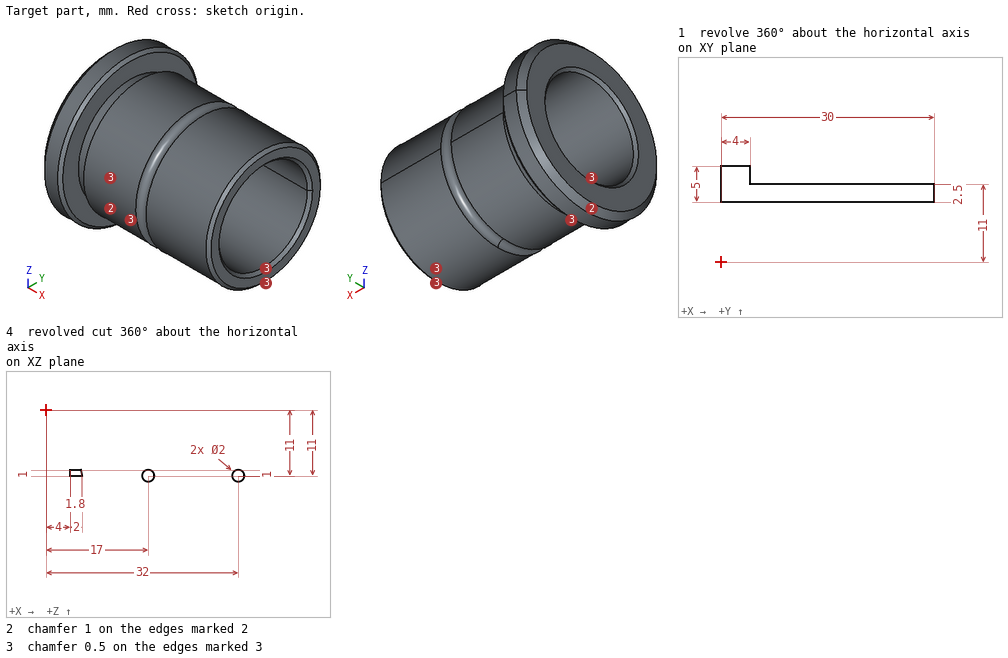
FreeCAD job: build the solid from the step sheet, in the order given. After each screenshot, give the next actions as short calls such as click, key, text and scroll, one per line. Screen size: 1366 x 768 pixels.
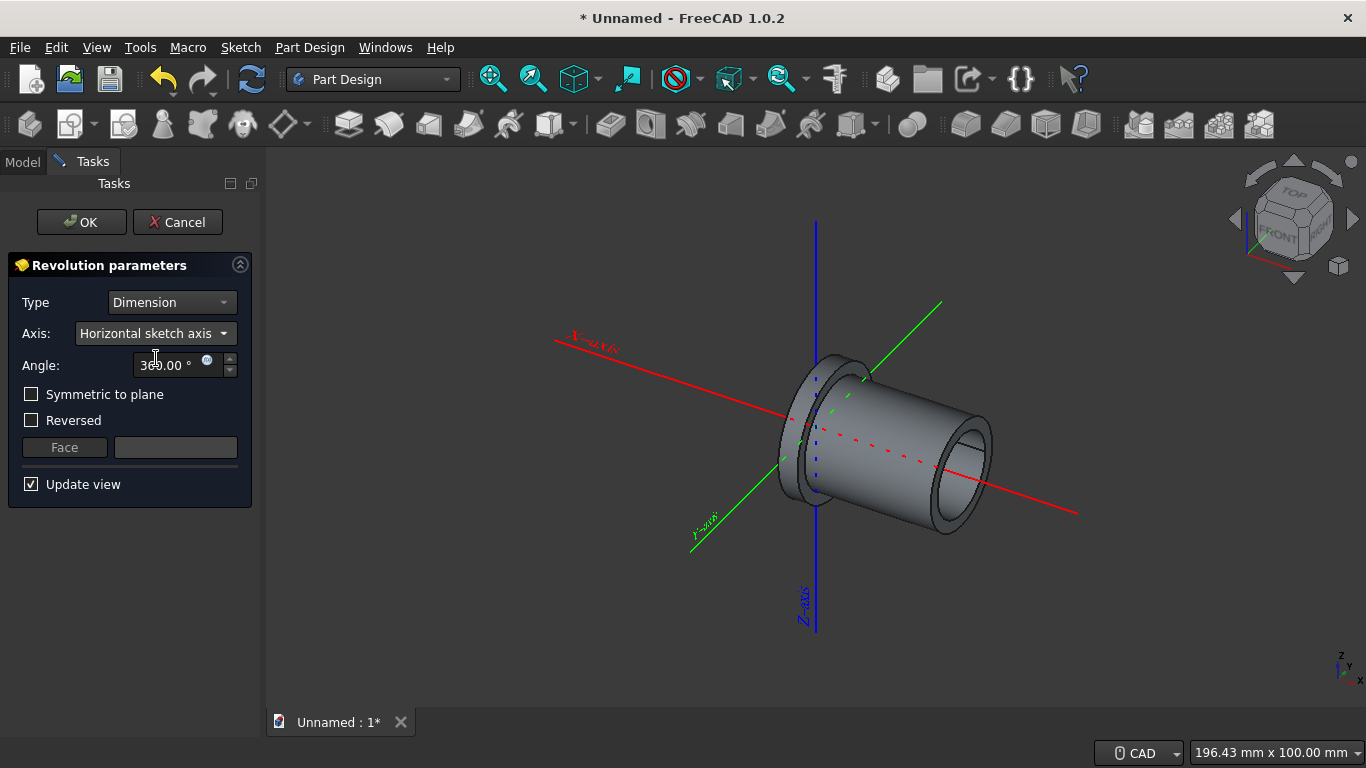
click(82, 222)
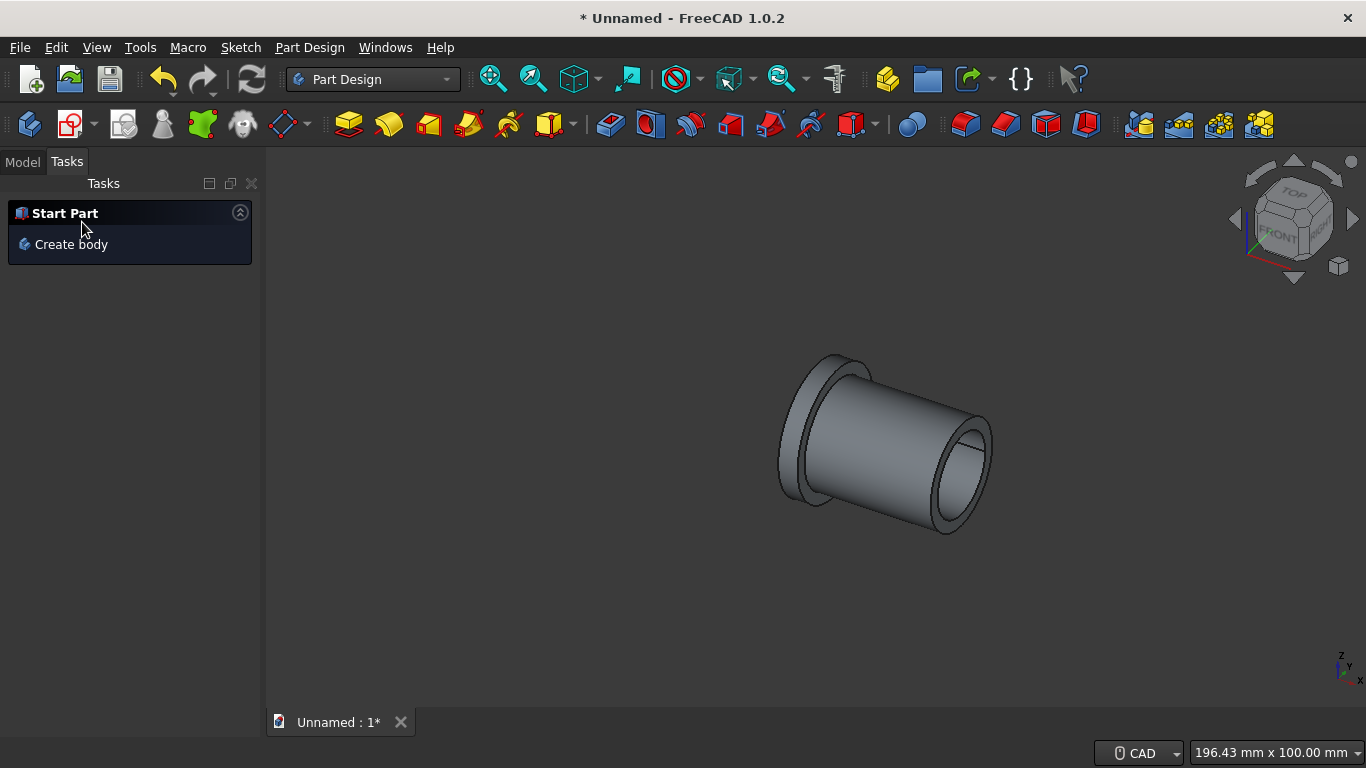
click(494, 80)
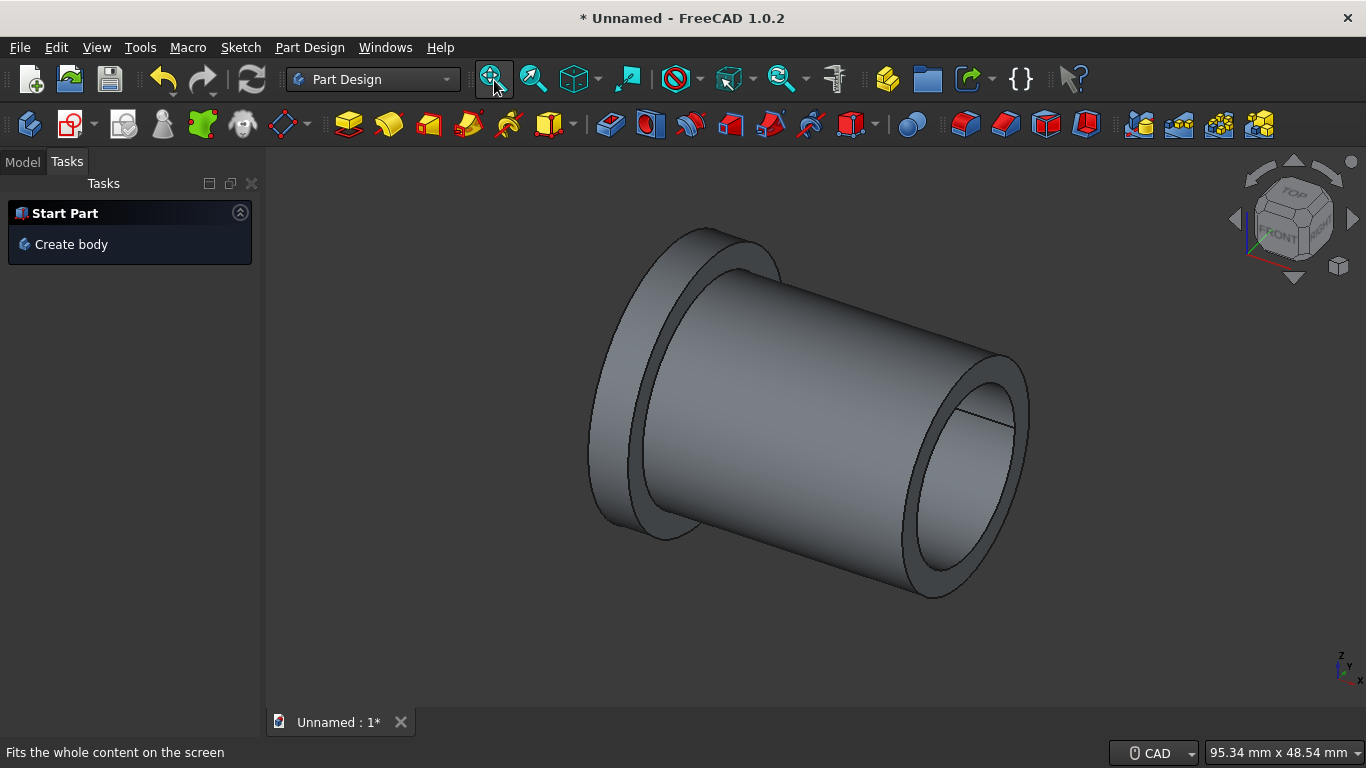
click(690, 231)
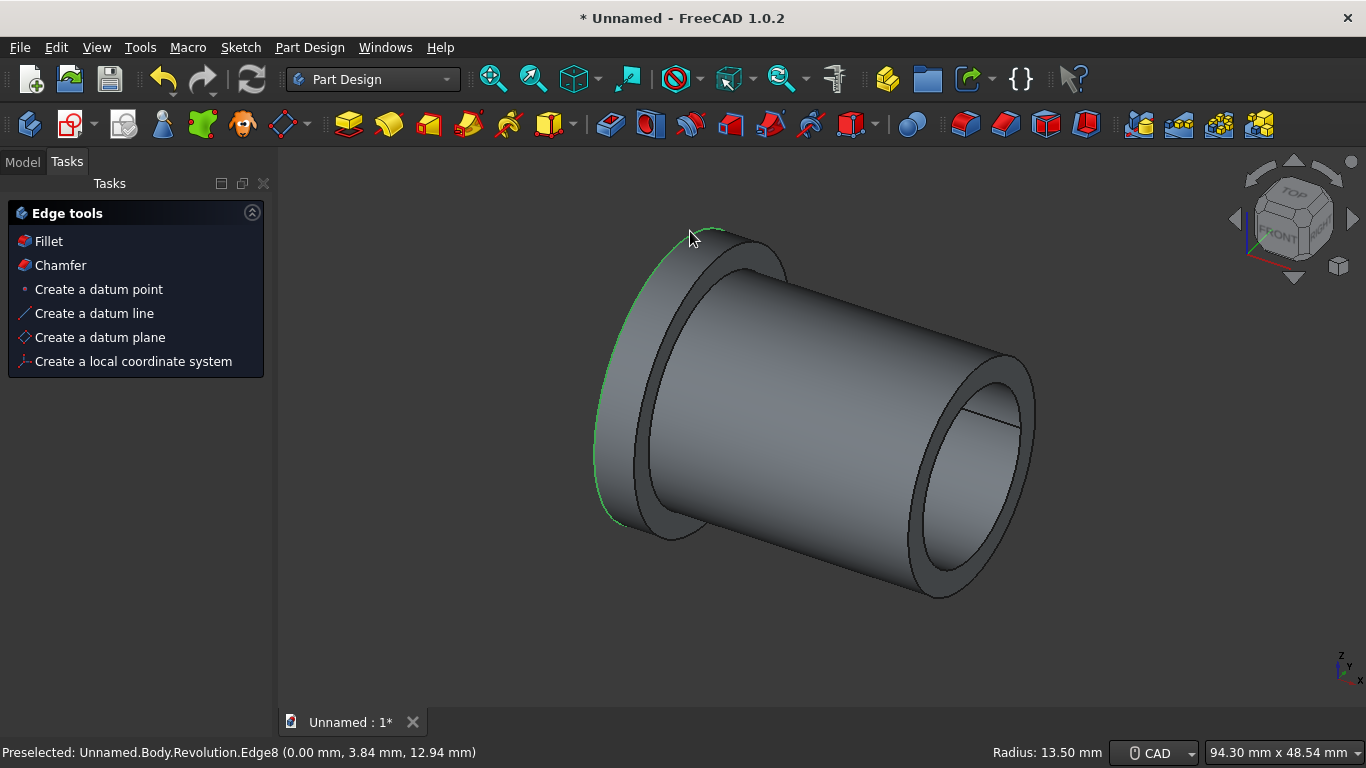
click(1006, 124)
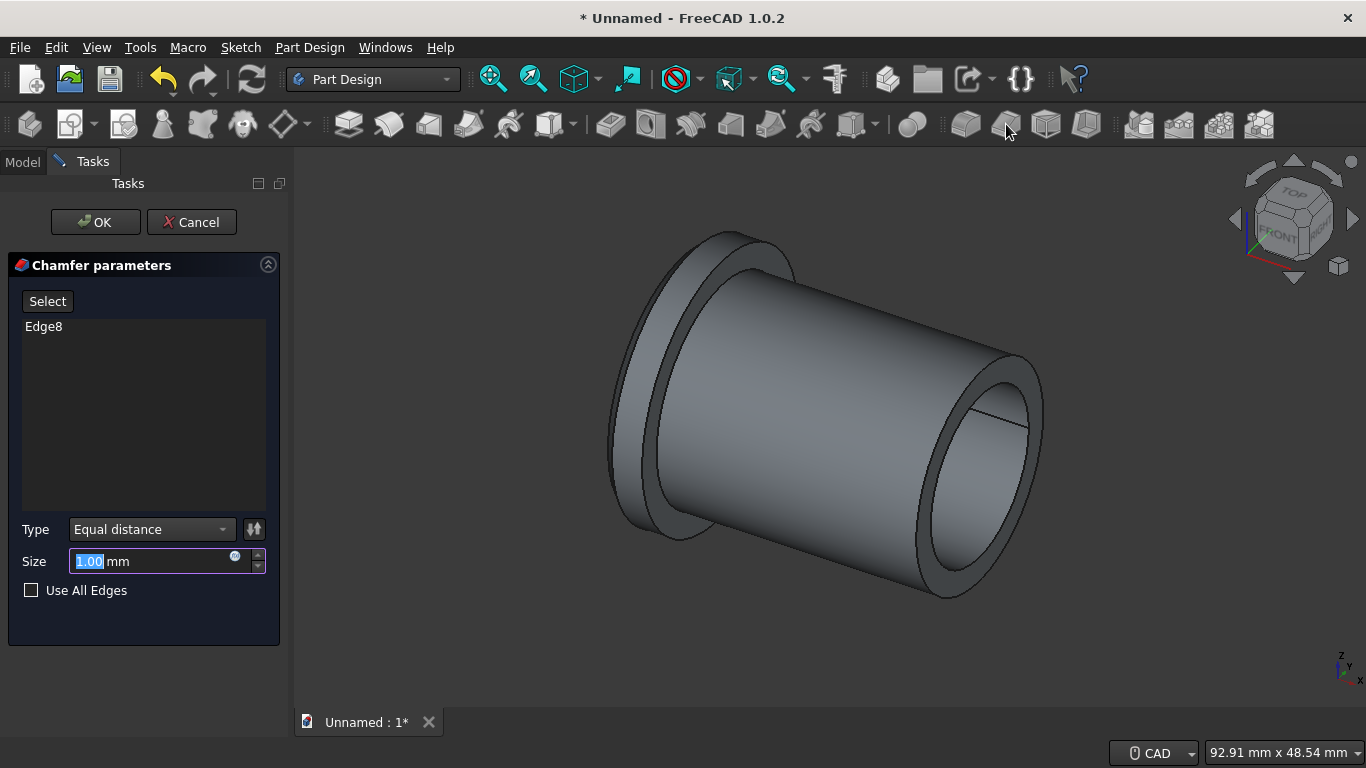
text(1)
key(Tab)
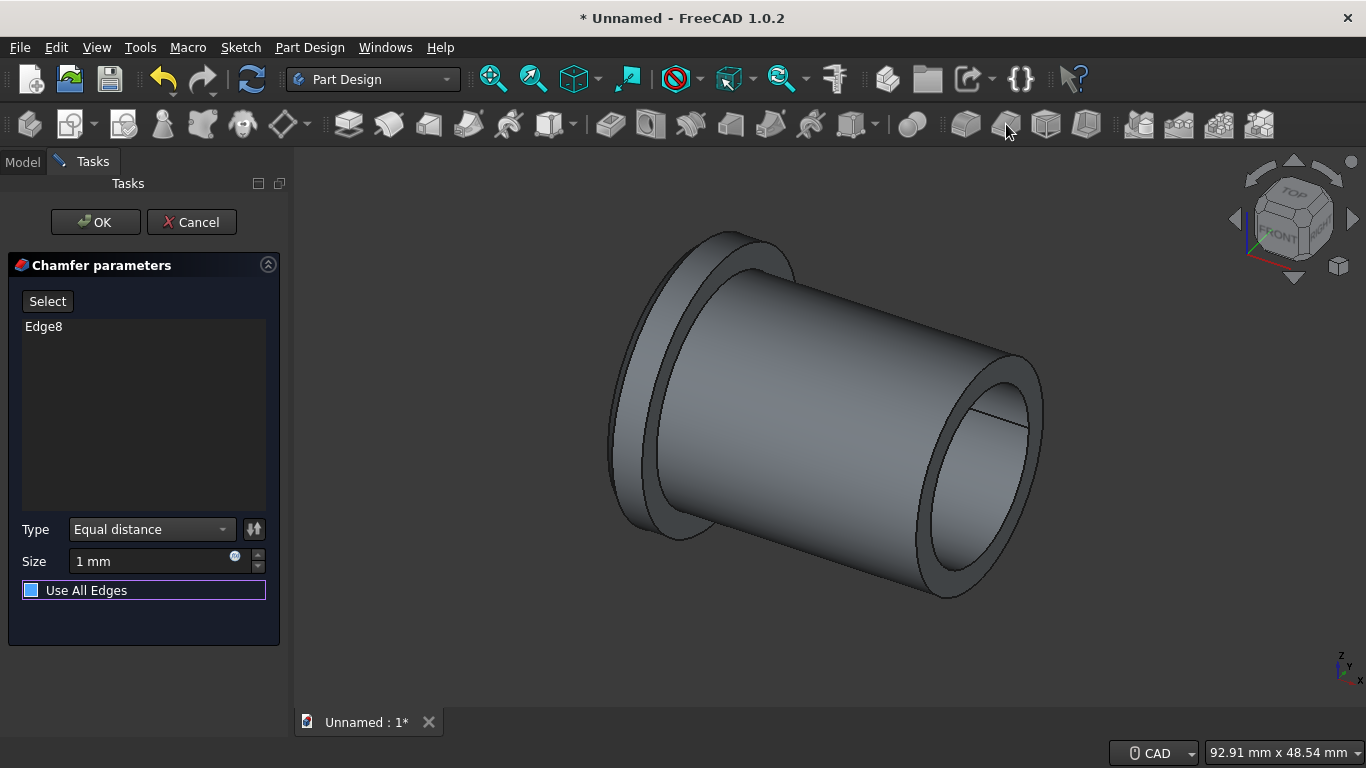
click(96, 222)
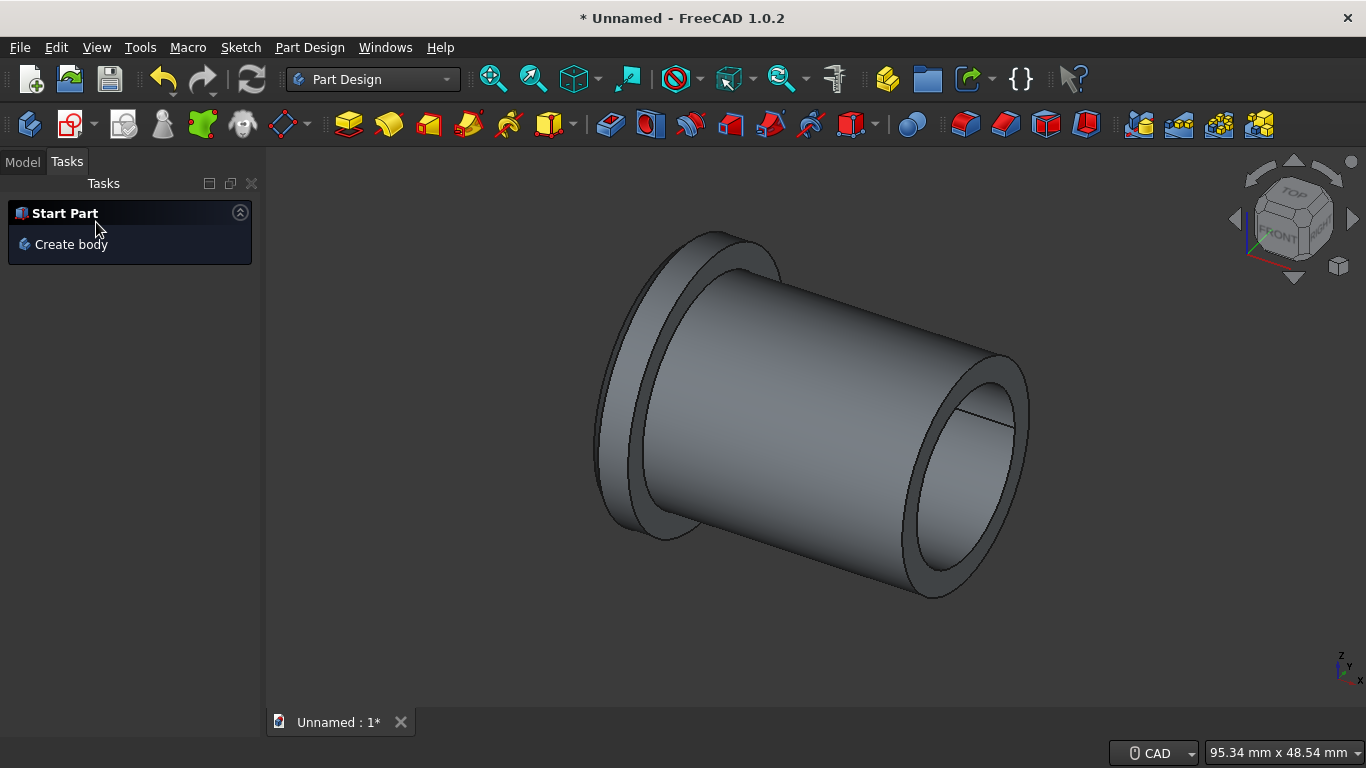
click(902, 539)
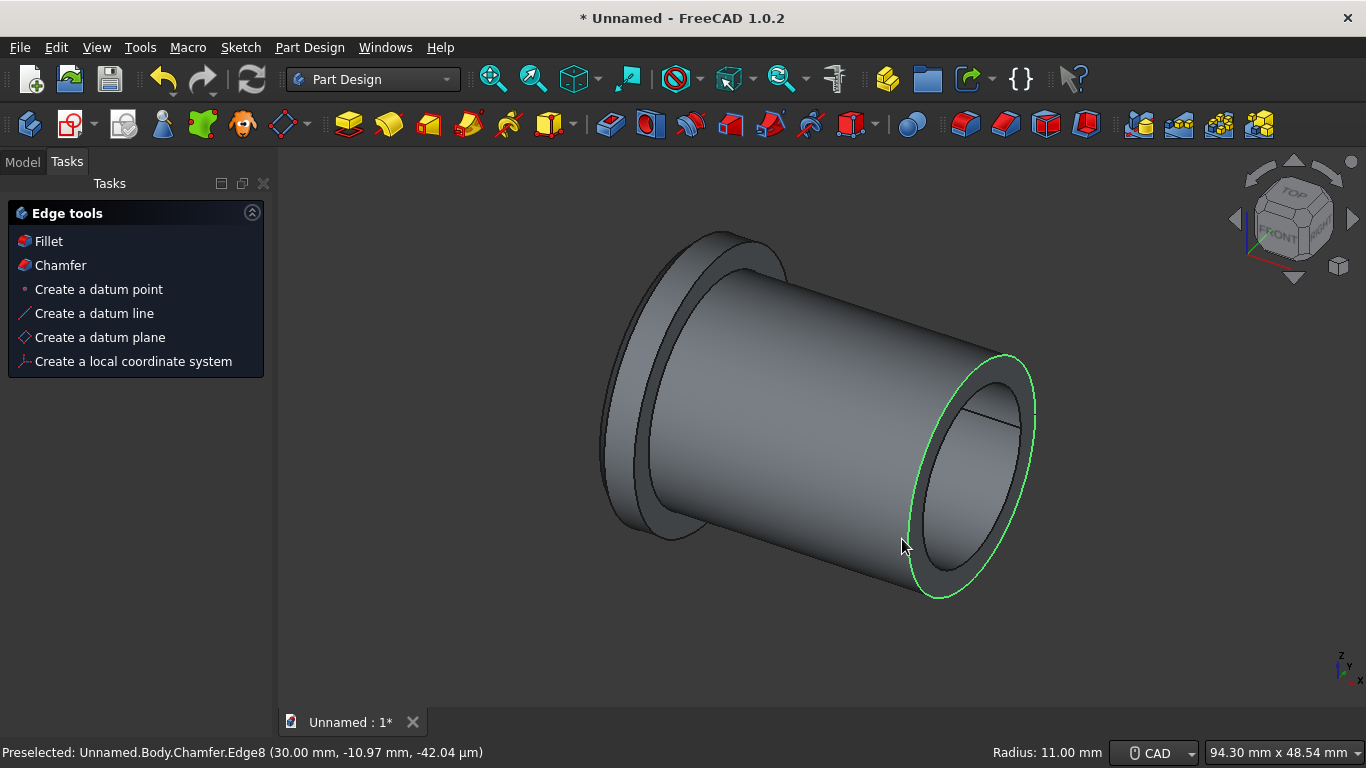
click(634, 467, ctrl)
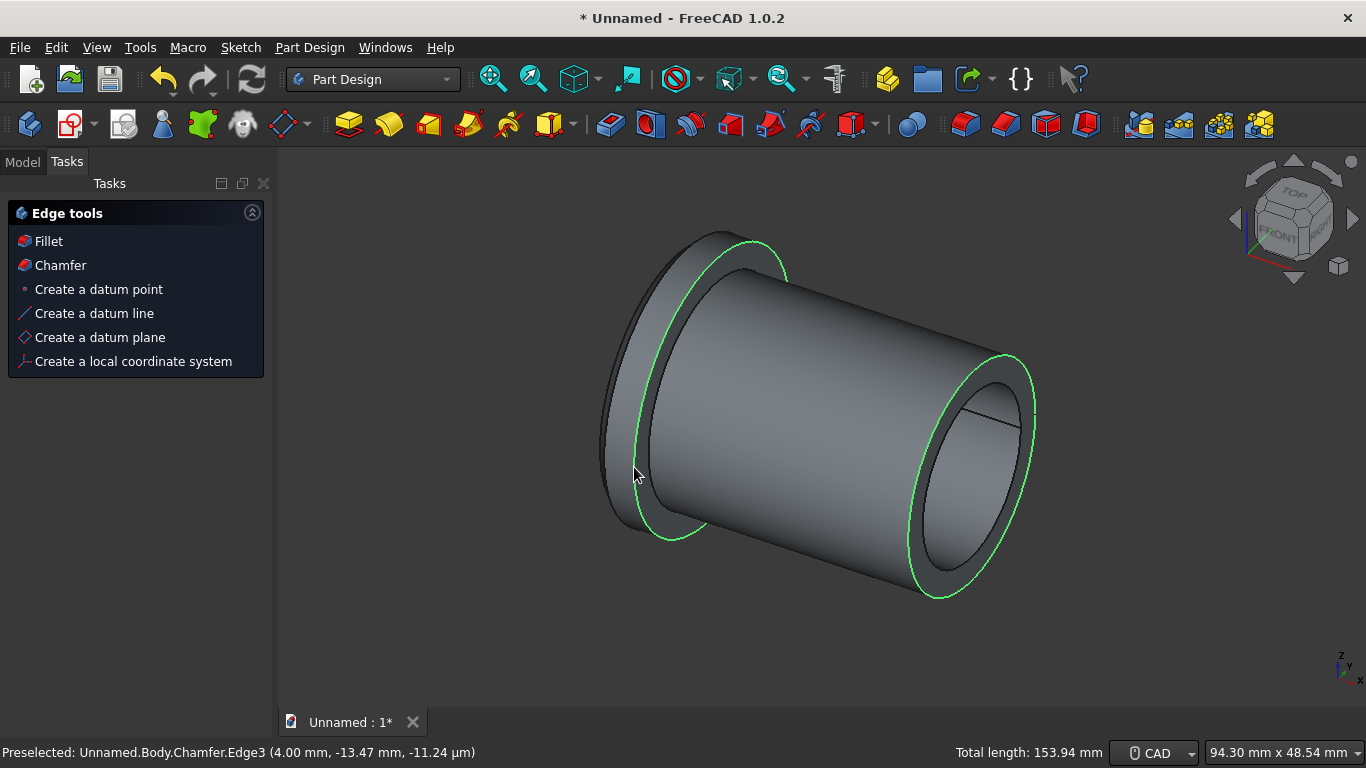
click(957, 567, ctrl)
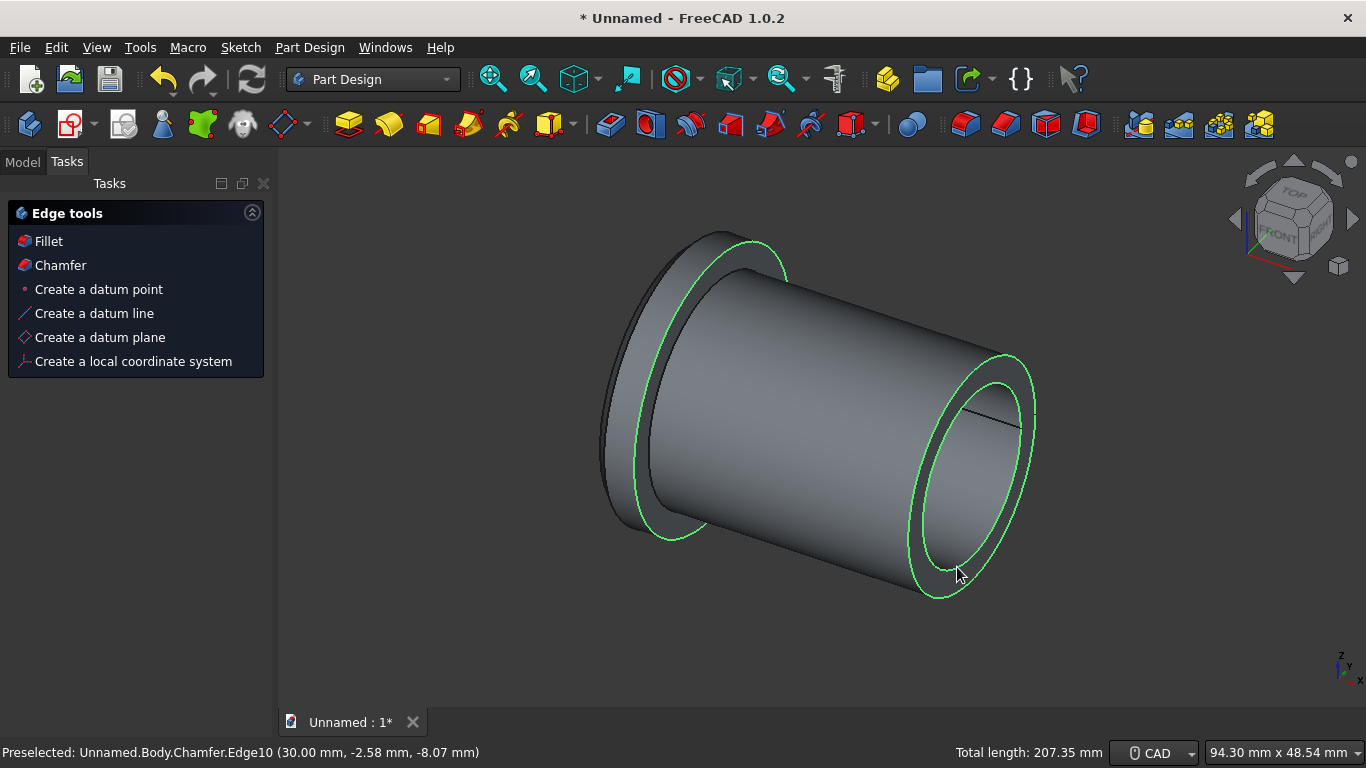
key(0)